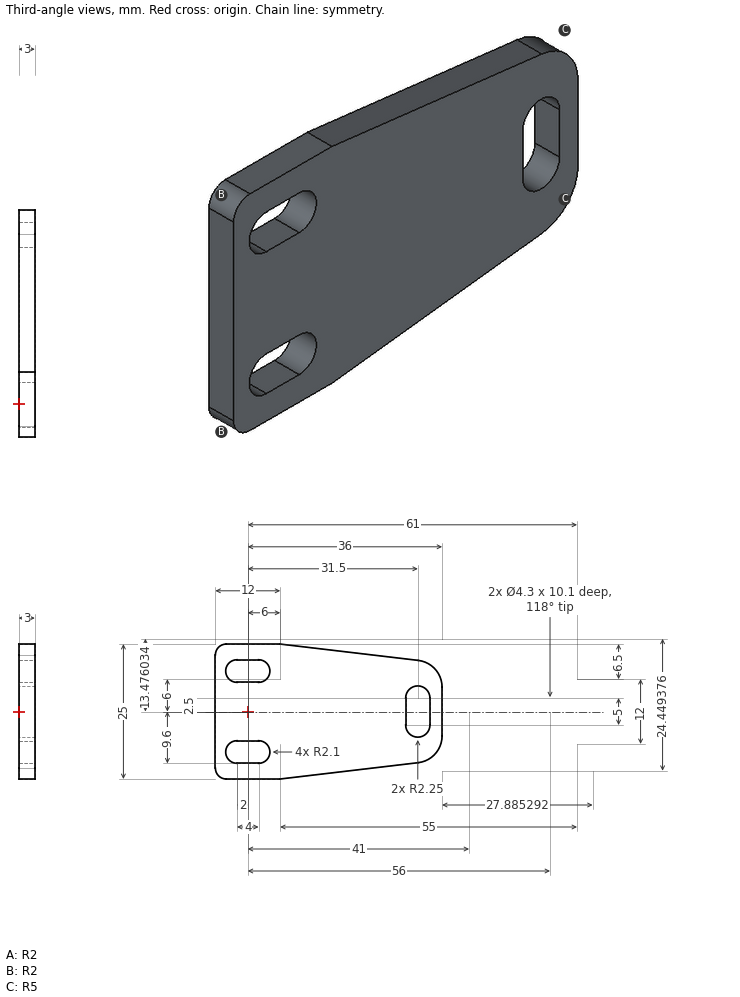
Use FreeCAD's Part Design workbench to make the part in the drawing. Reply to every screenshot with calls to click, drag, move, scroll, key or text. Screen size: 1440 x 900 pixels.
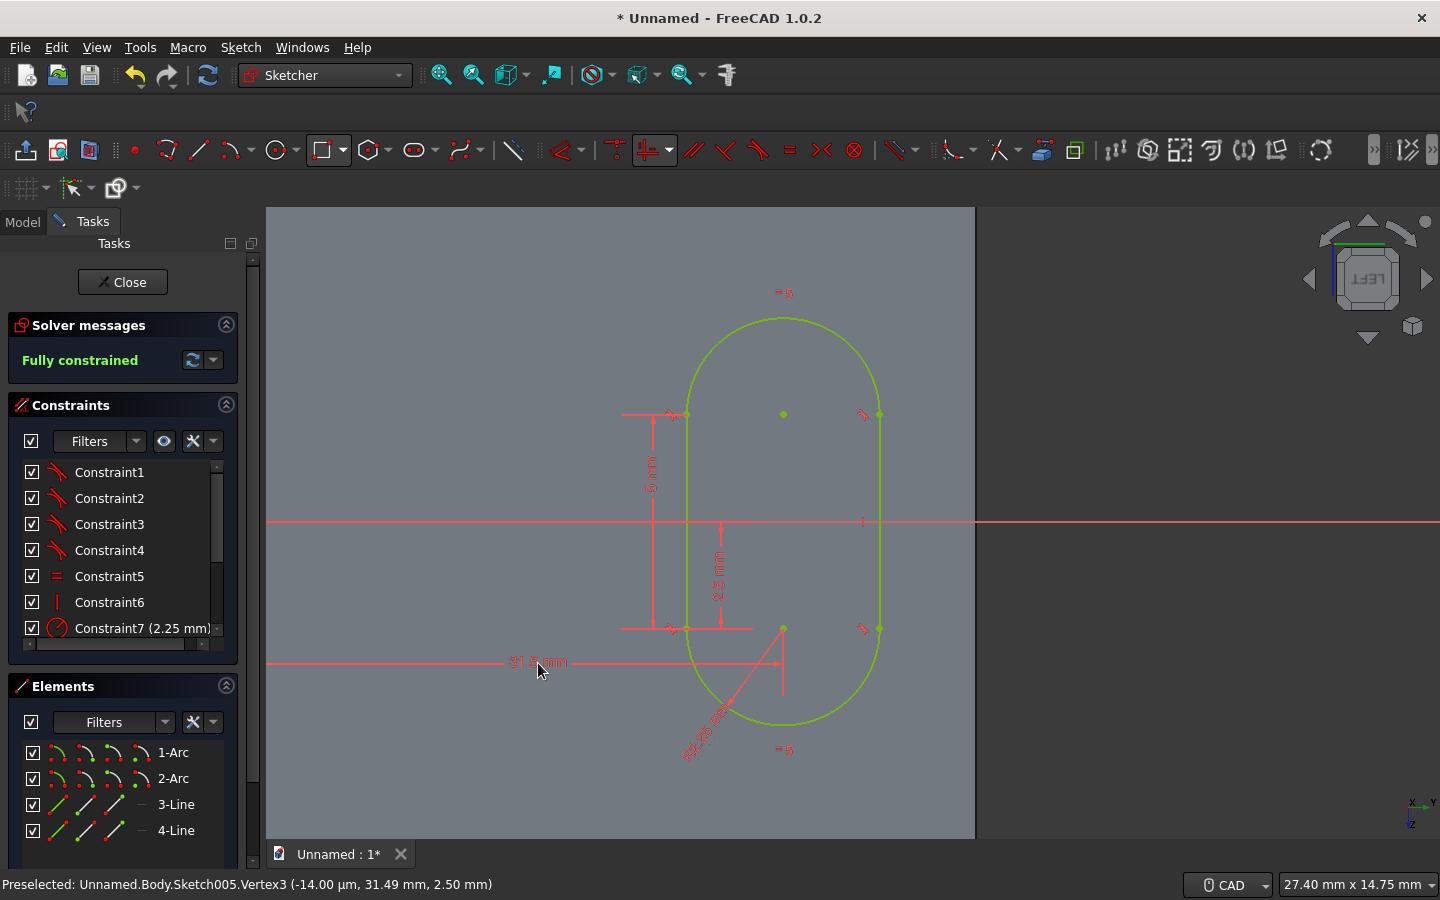
click(123, 282)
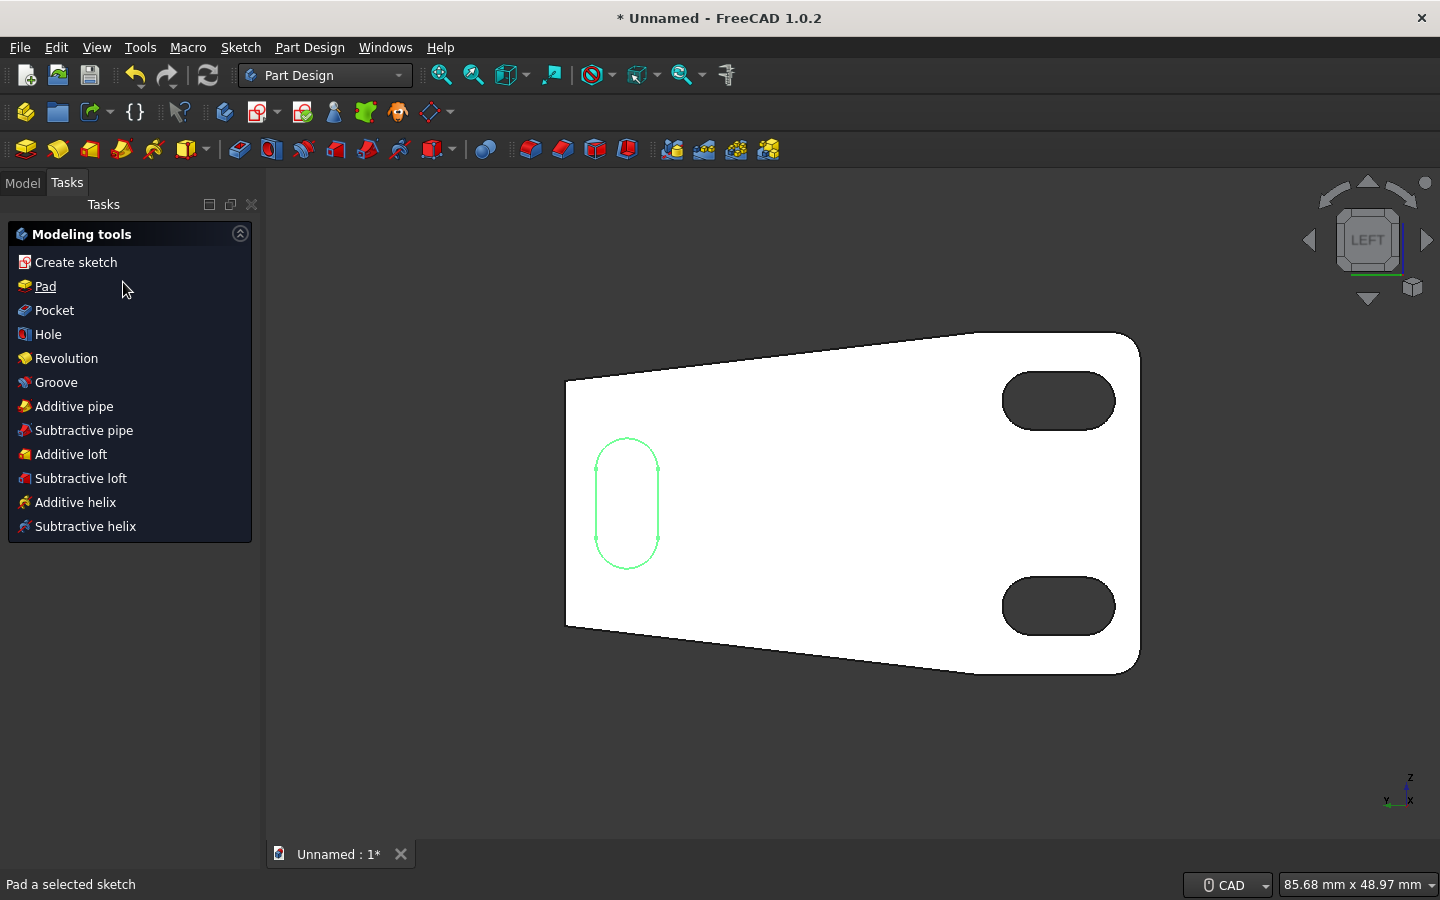
click(240, 150)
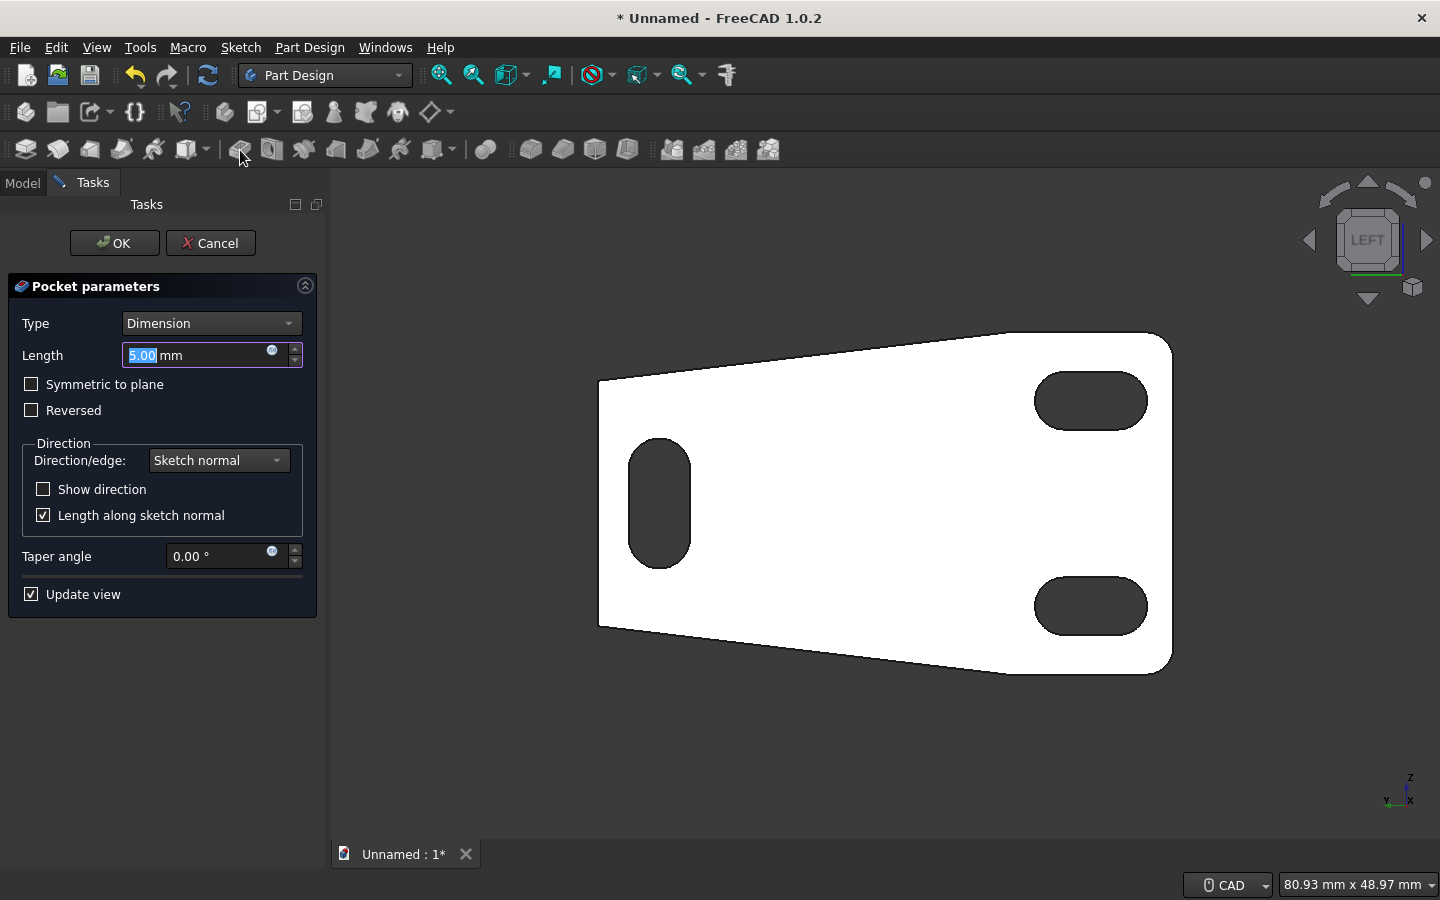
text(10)
key(Tab)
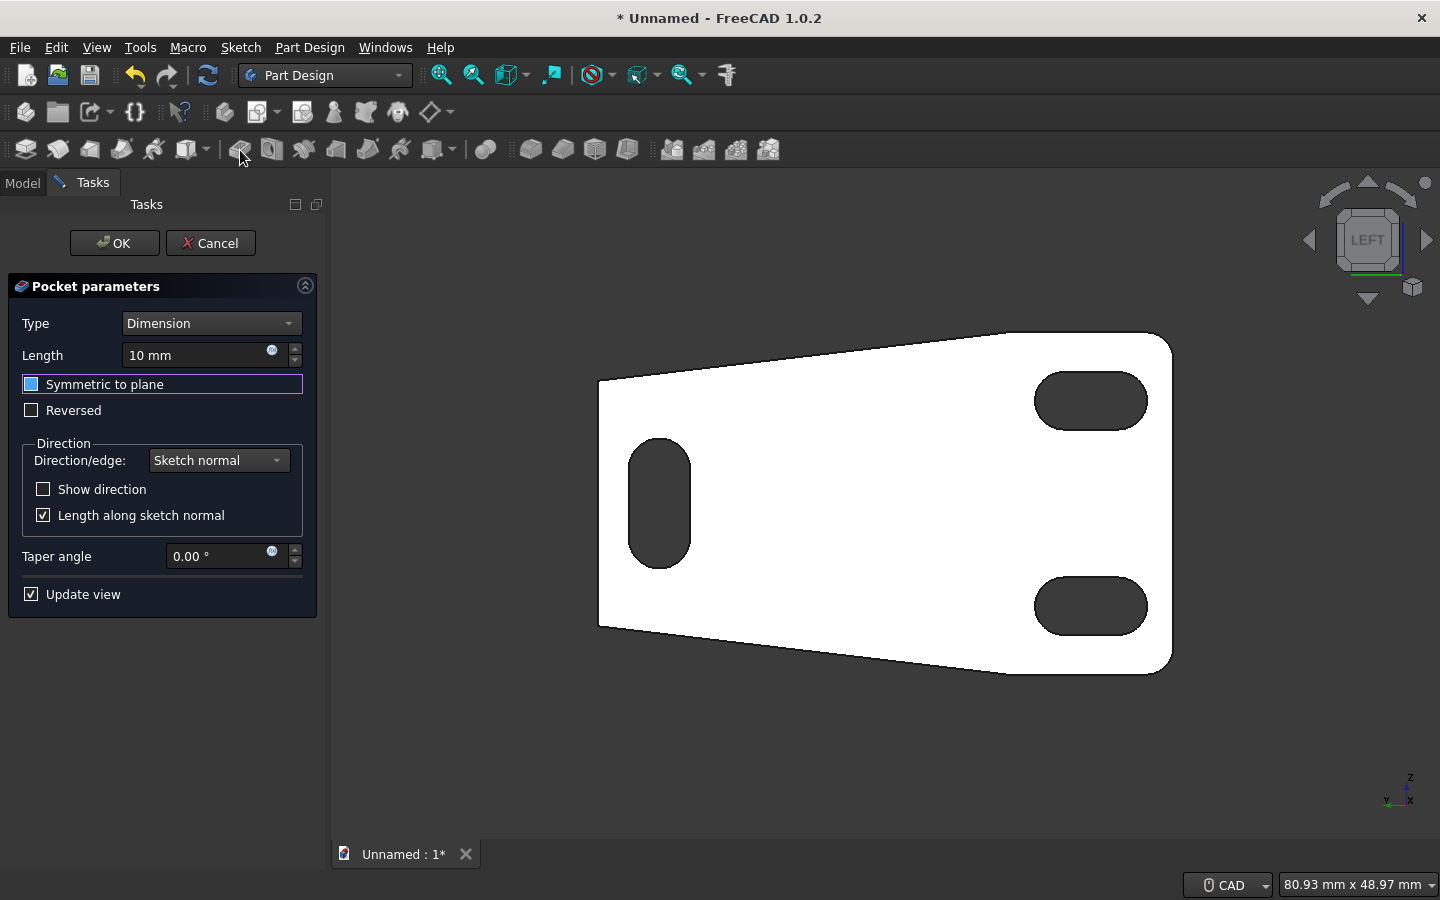
click(115, 243)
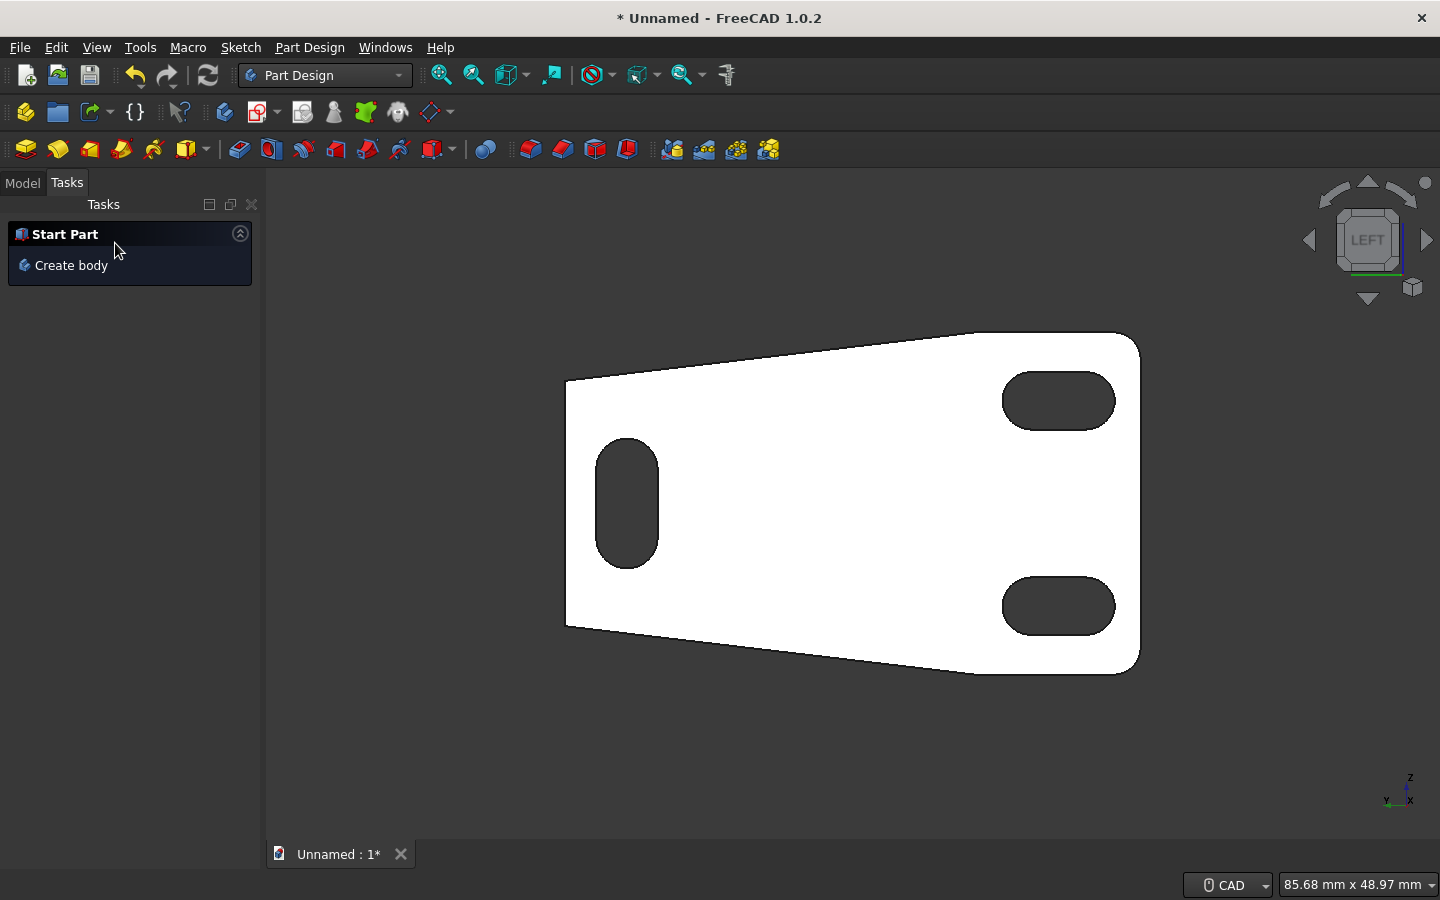
key(0)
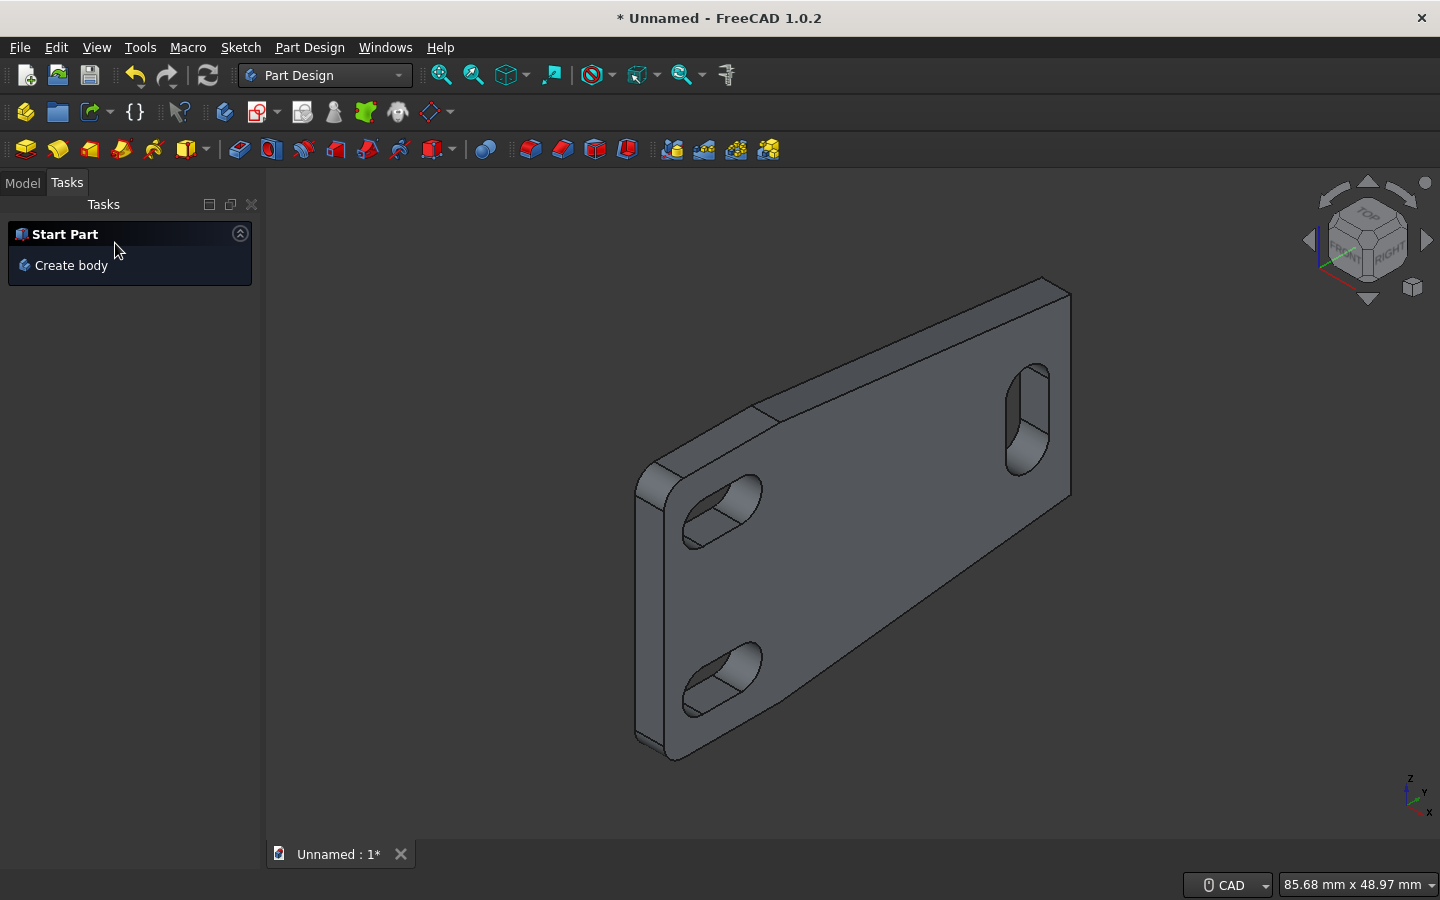
key(2)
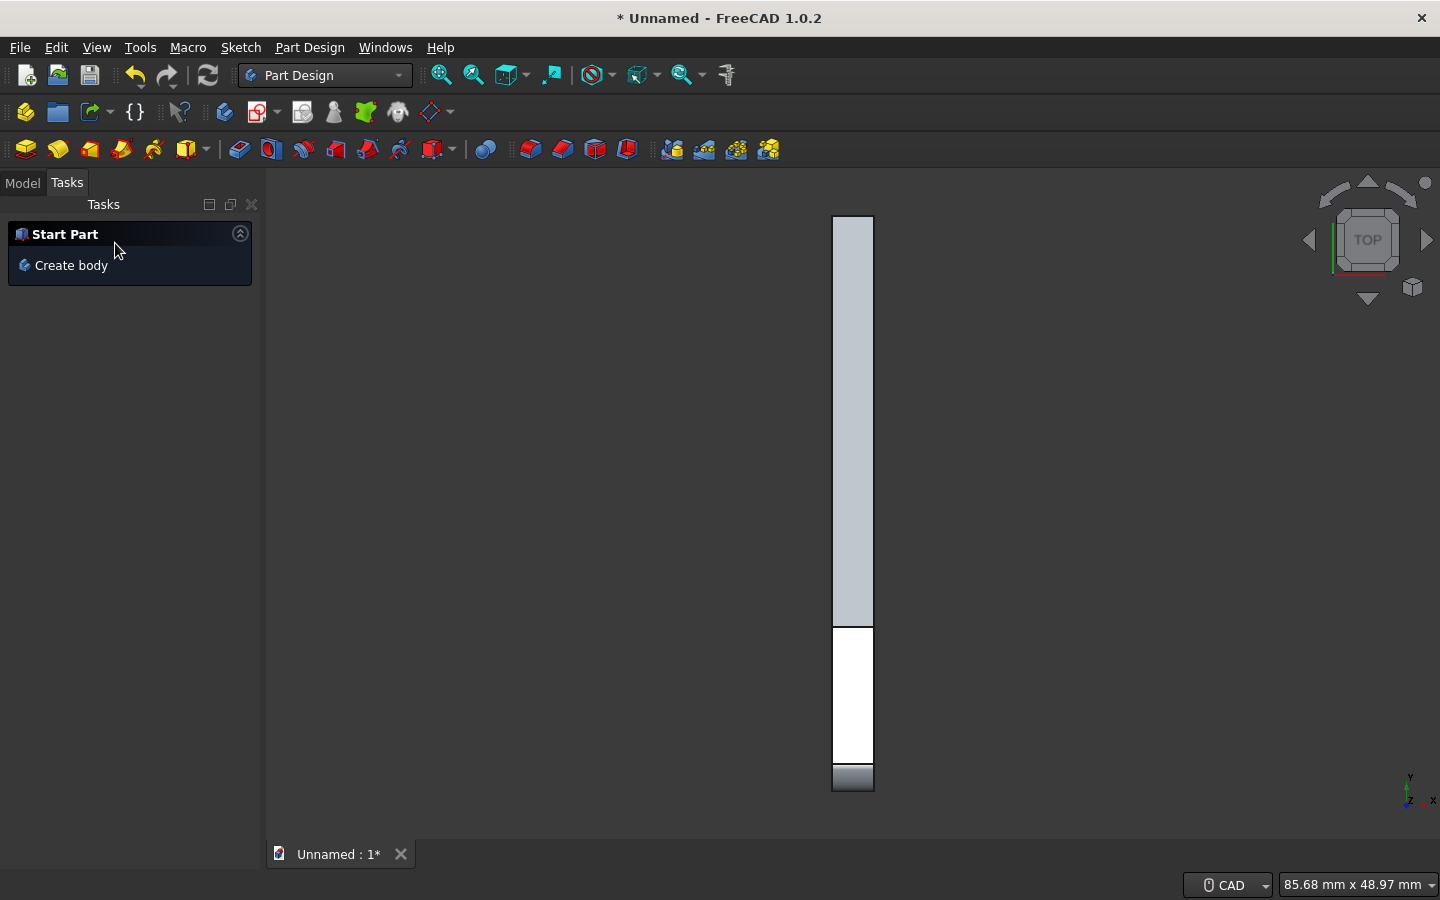
key(1)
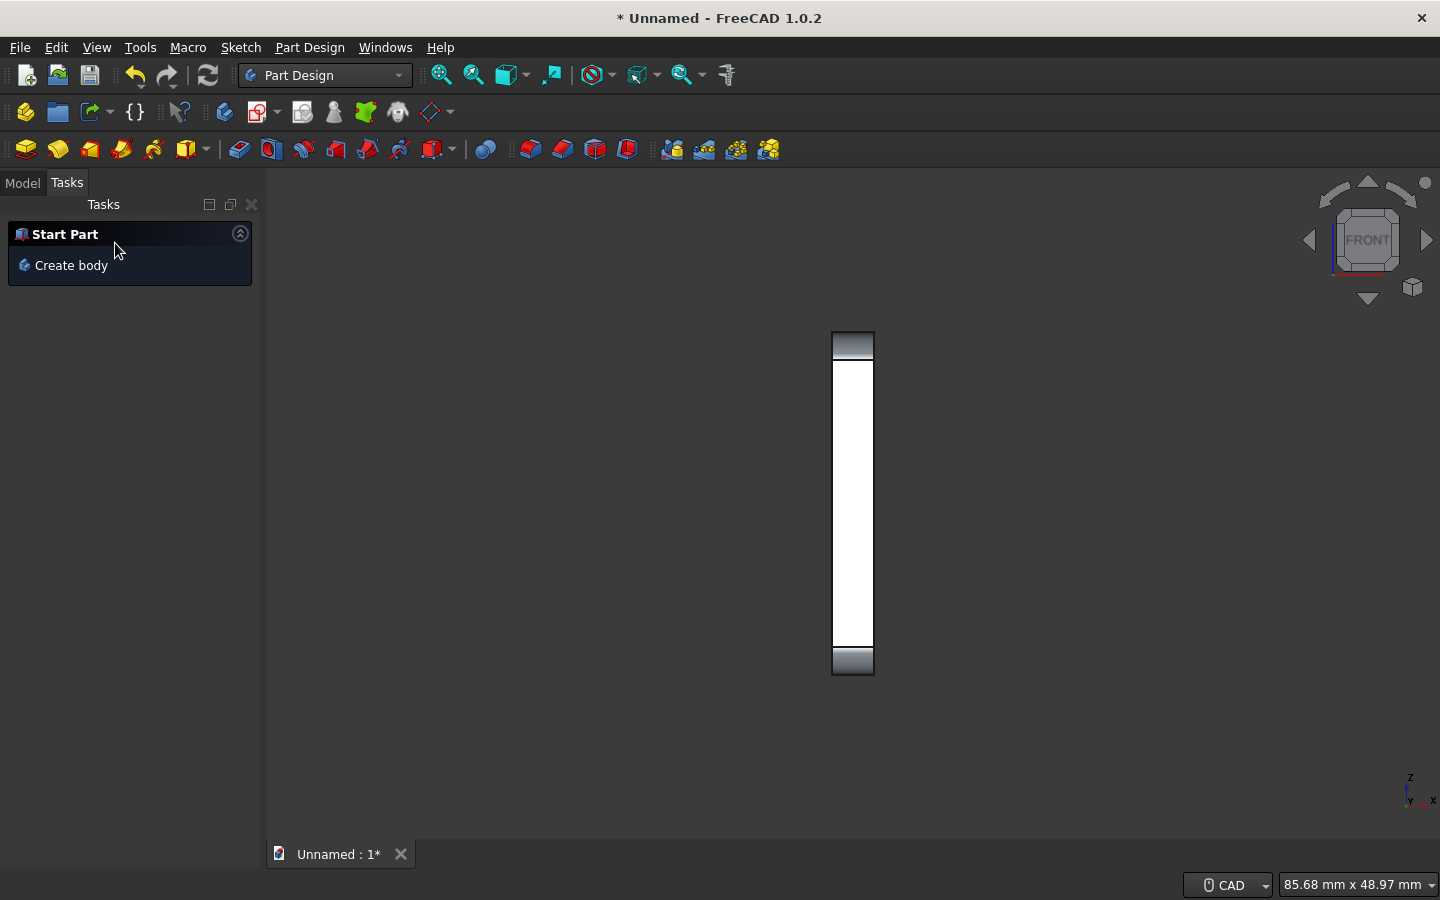
key(3)